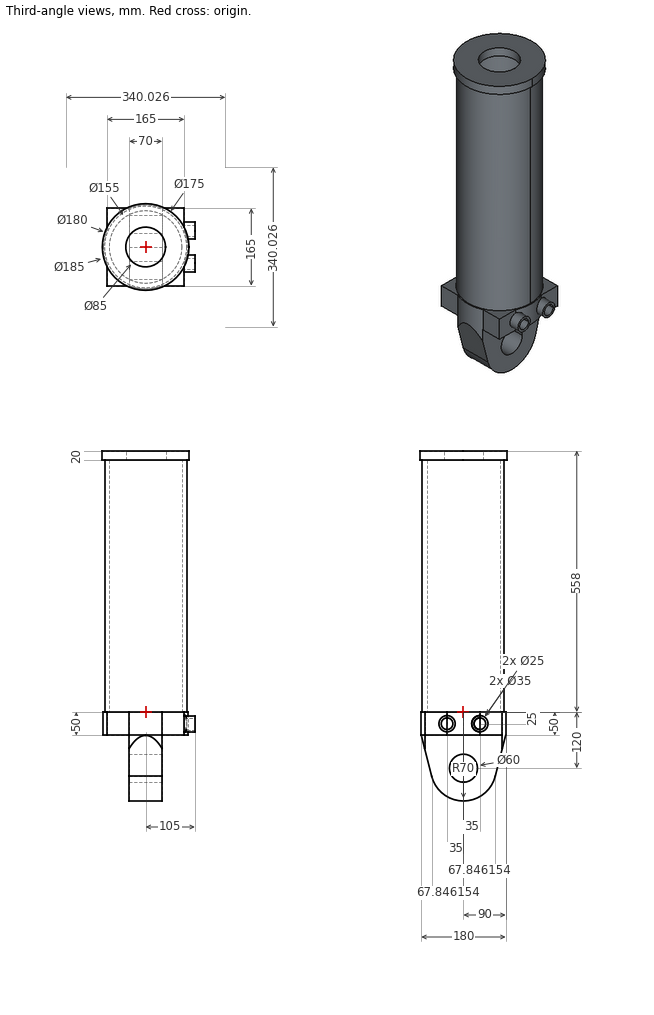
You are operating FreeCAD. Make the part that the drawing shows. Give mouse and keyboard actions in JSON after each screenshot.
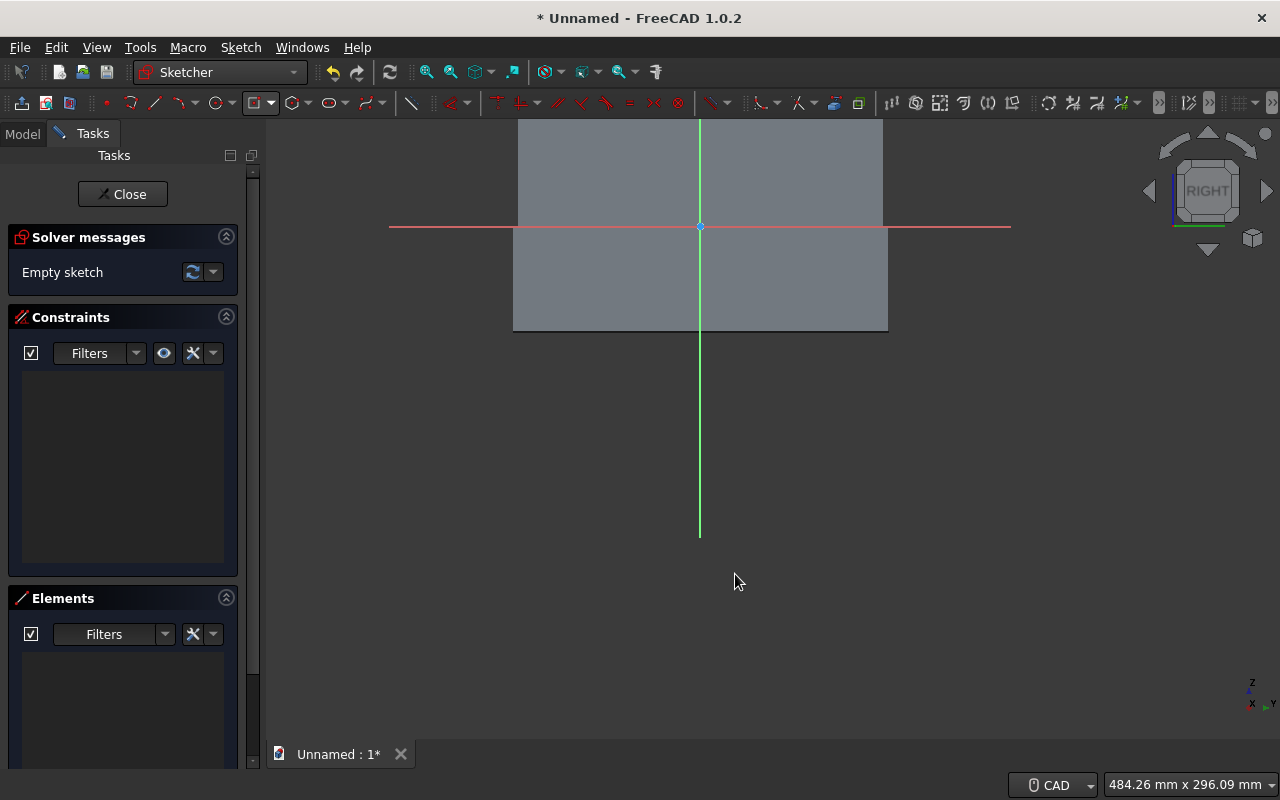
{"action": "left_click", "coordinate": [132, 104]}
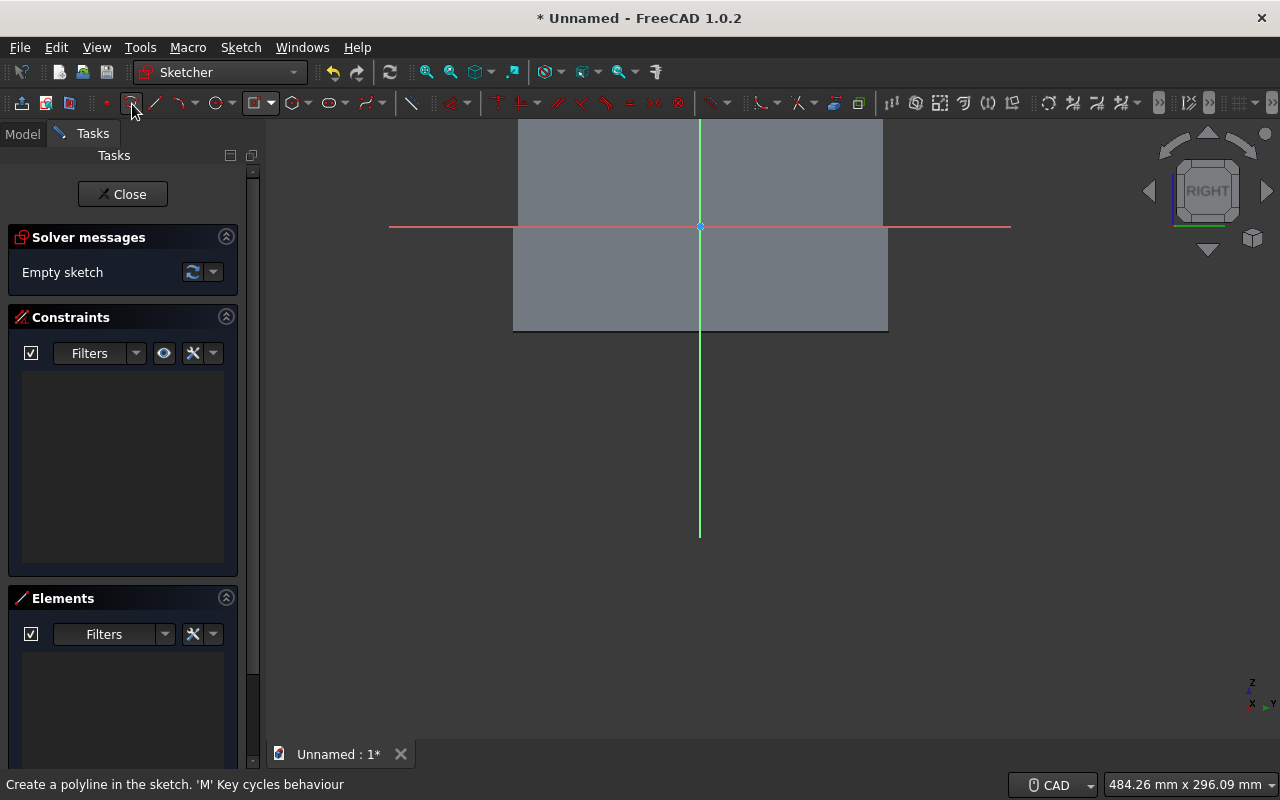
{"action": "left_click", "coordinate": [842, 514]}
{"action": "left_click", "coordinate": [889, 332]}
{"action": "left_click", "coordinate": [512, 332]}
{"action": "left_click", "coordinate": [558, 514]}
{"action": "right_click", "coordinate": [558, 514]}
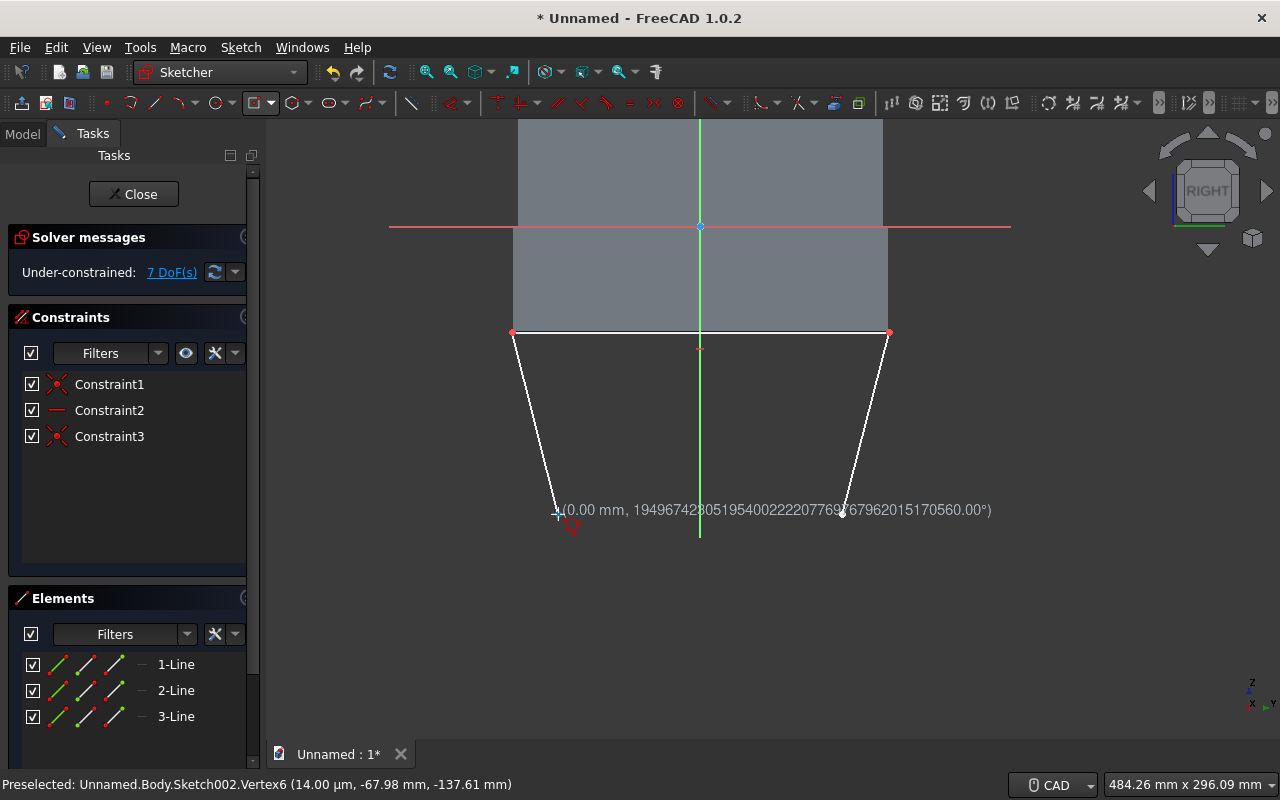
{"action": "left_click", "coordinate": [180, 104]}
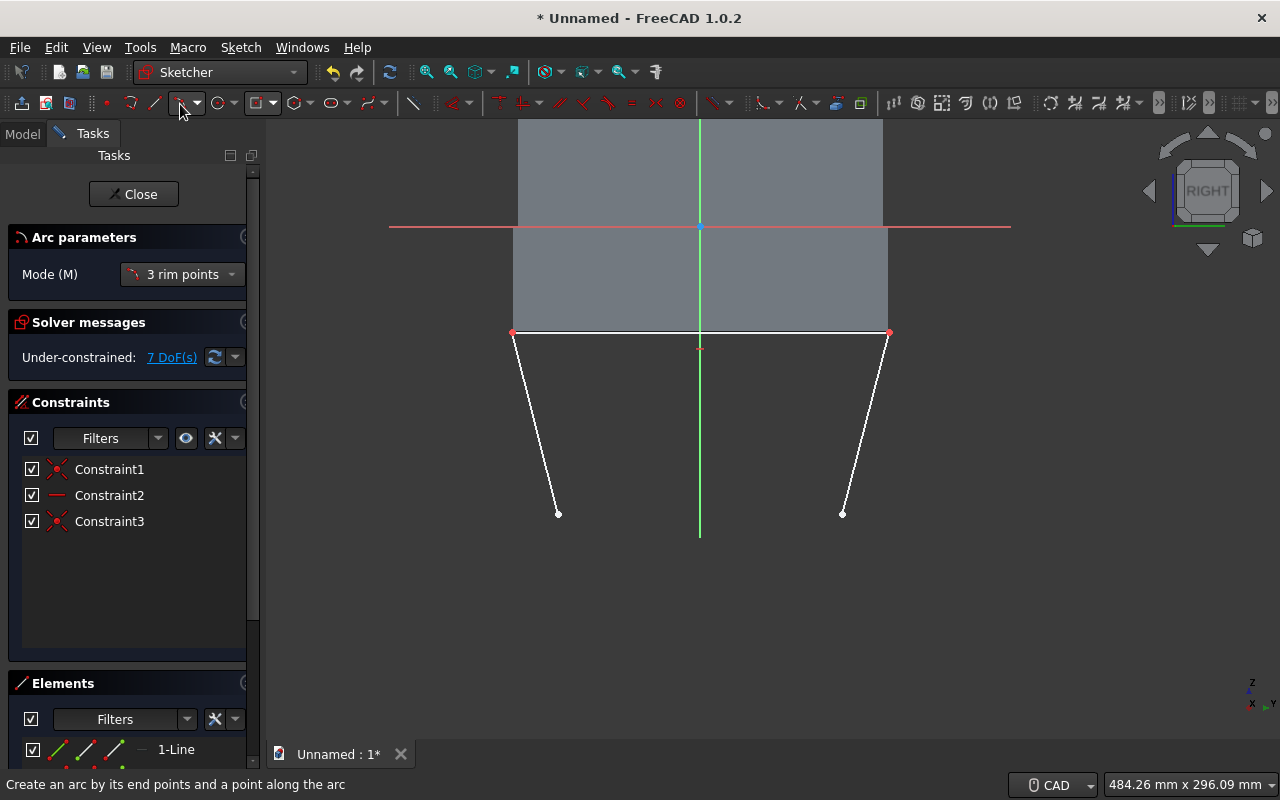
{"action": "left_click", "coordinate": [558, 515]}
{"action": "left_click", "coordinate": [842, 515]}
{"action": "left_click", "coordinate": [662, 620]}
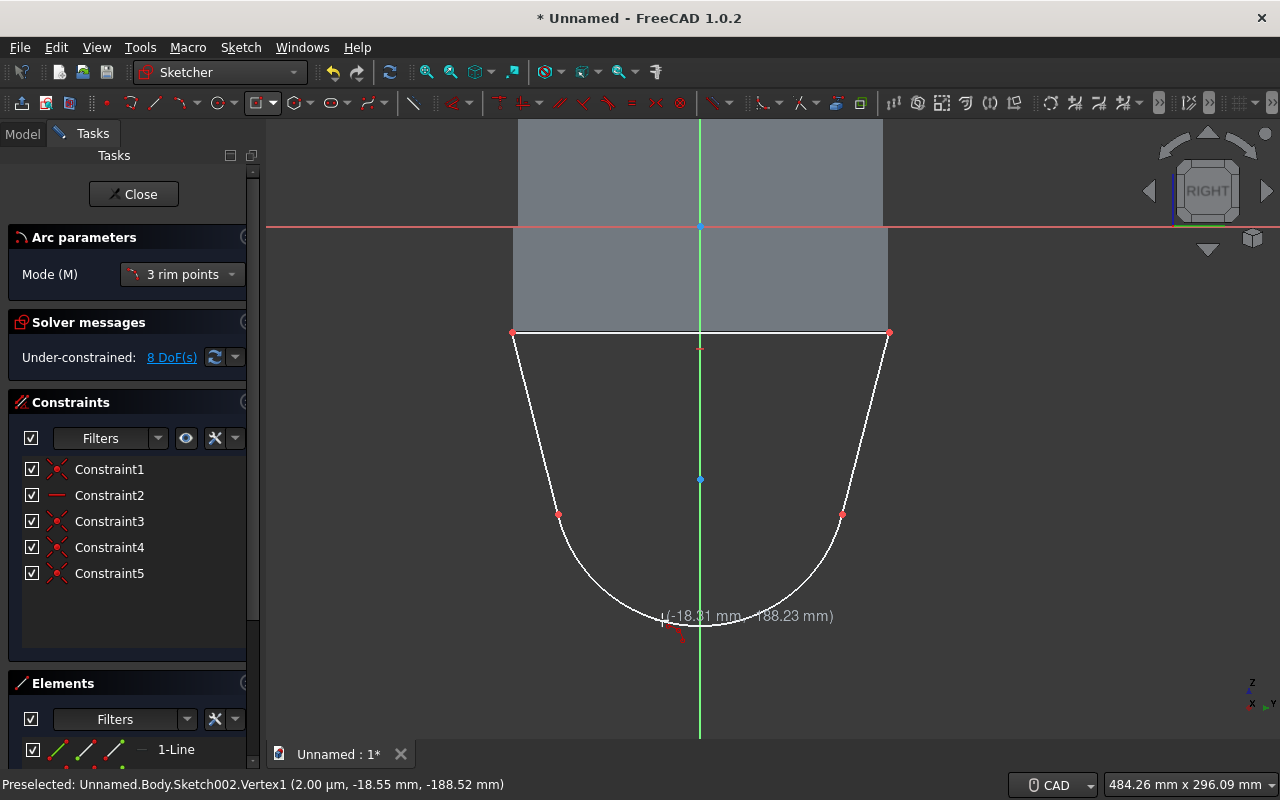
{"action": "key", "text": "g c"}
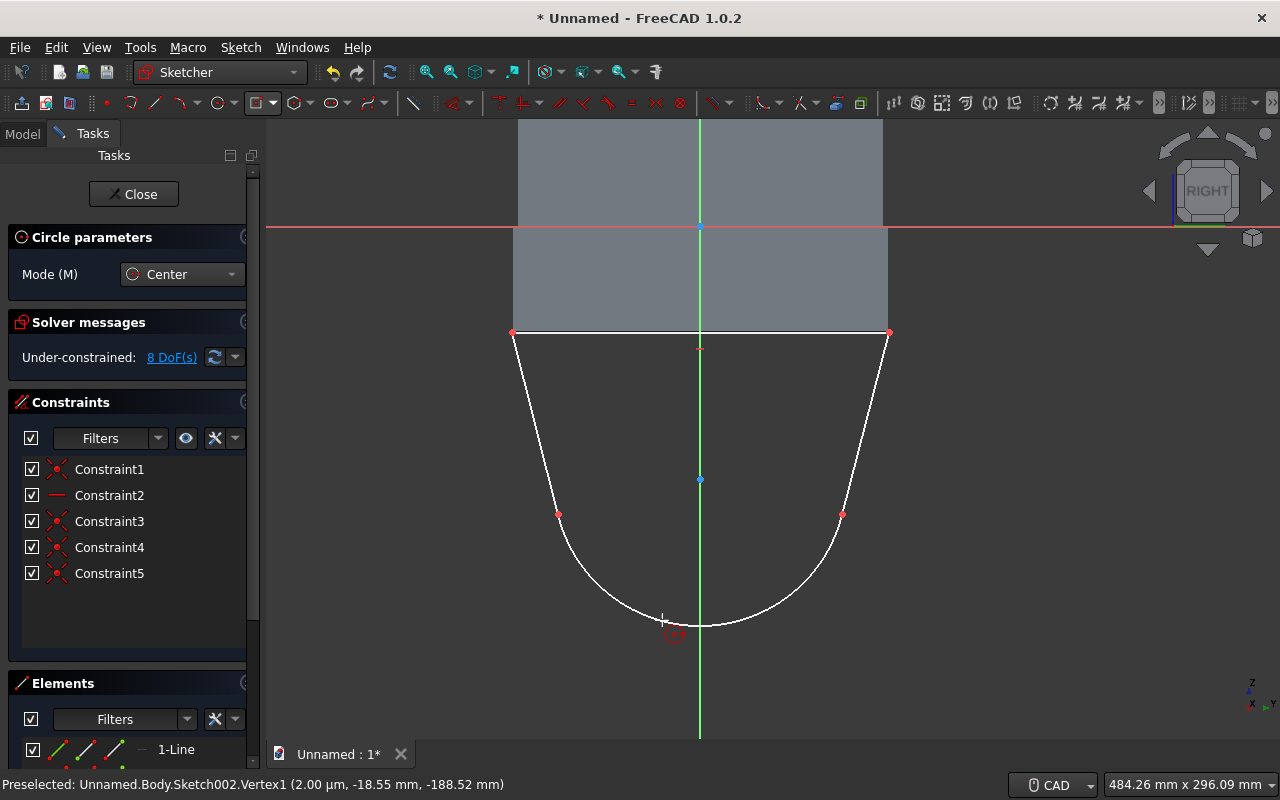
{"action": "left_click", "coordinate": [700, 478]}
{"action": "left_click", "coordinate": [745, 434]}
{"action": "key", "text": "Escape"}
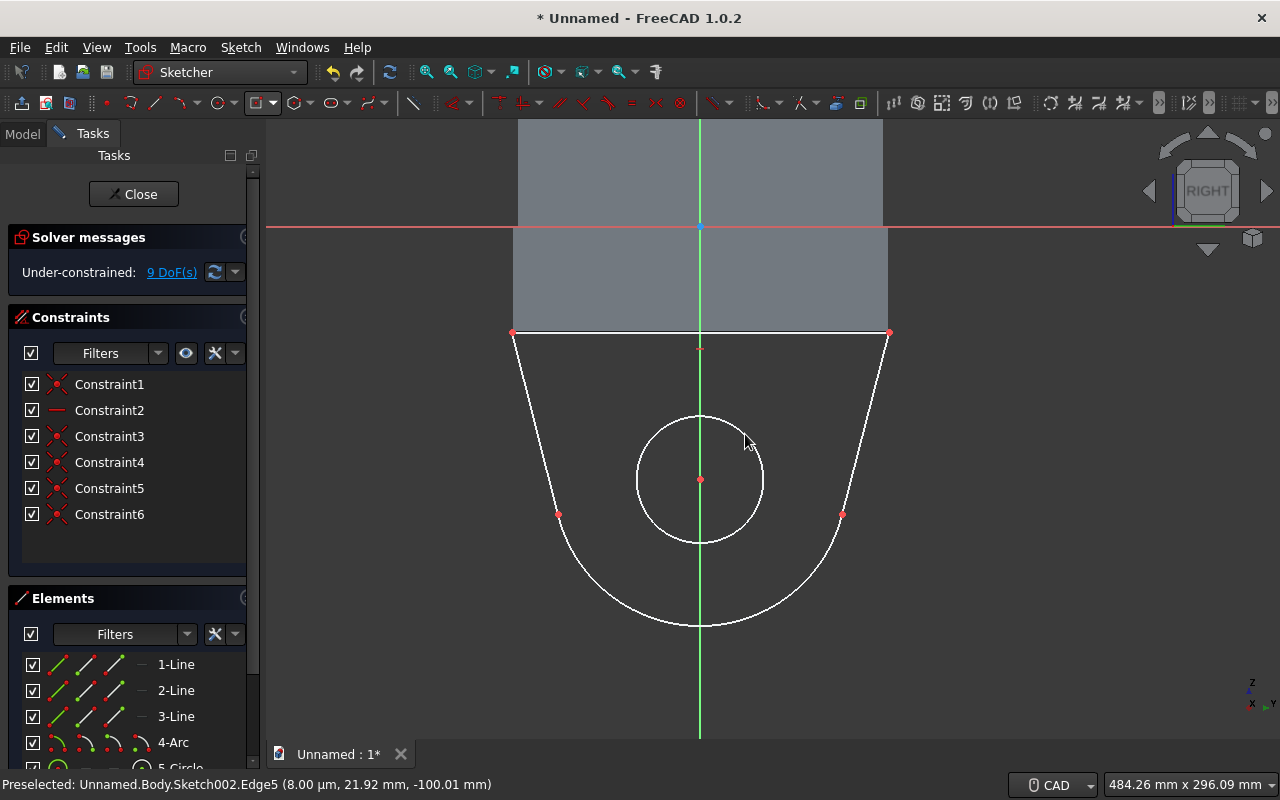
{"action": "left_click", "coordinate": [700, 480]}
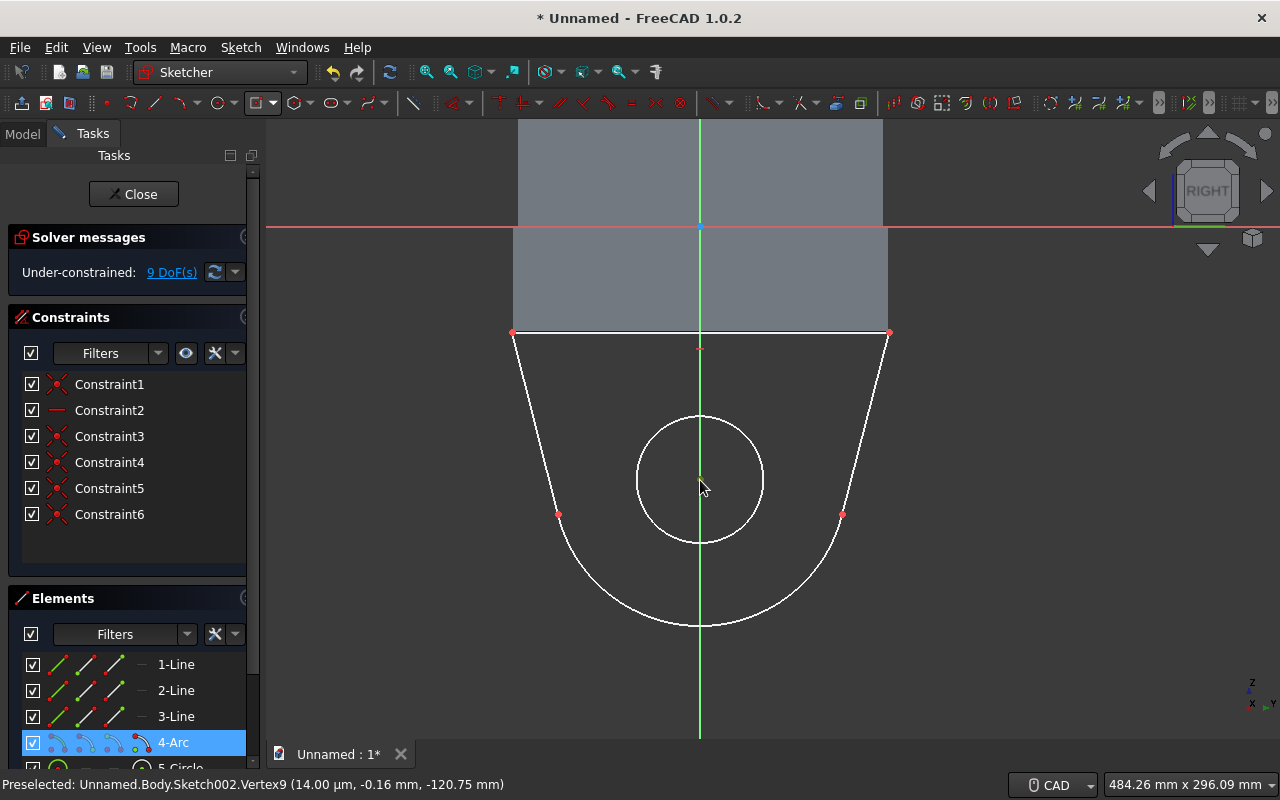
{"action": "left_click", "coordinate": [700, 671]}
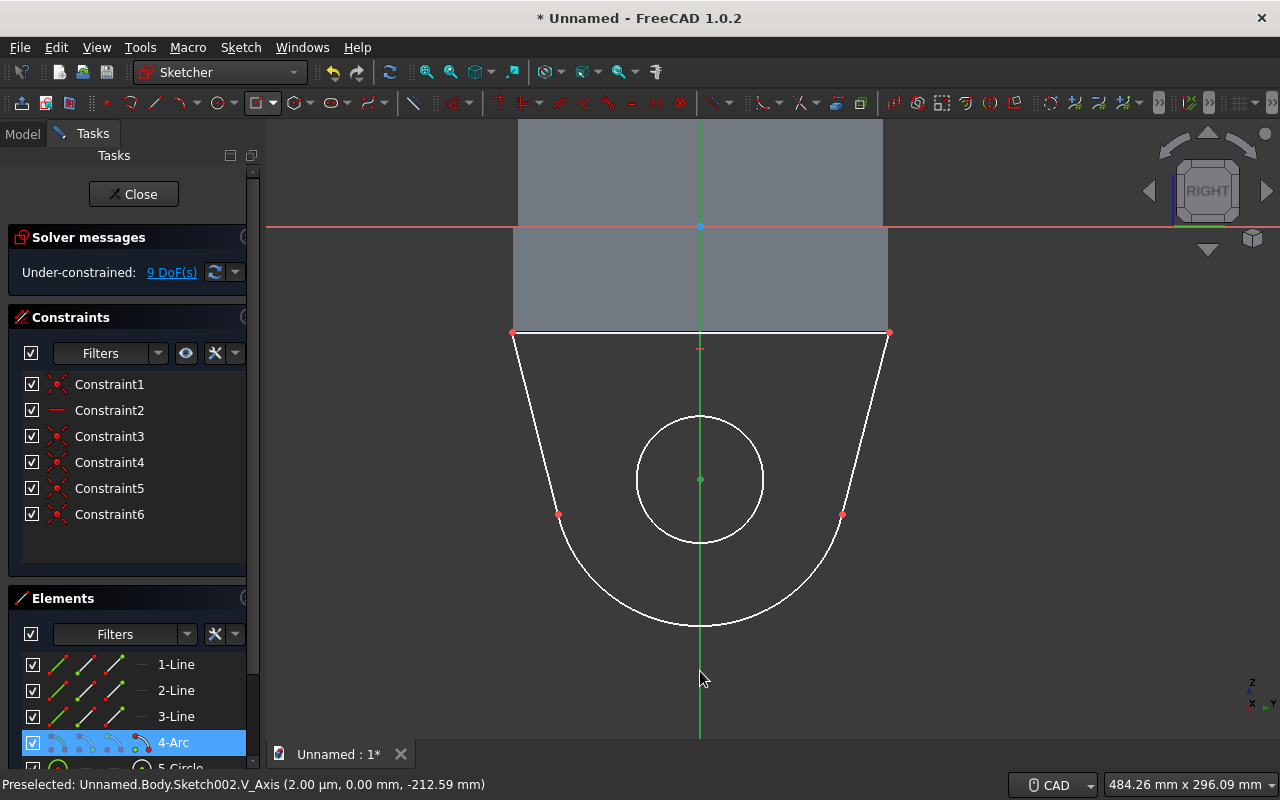
{"action": "left_click", "coordinate": [500, 104]}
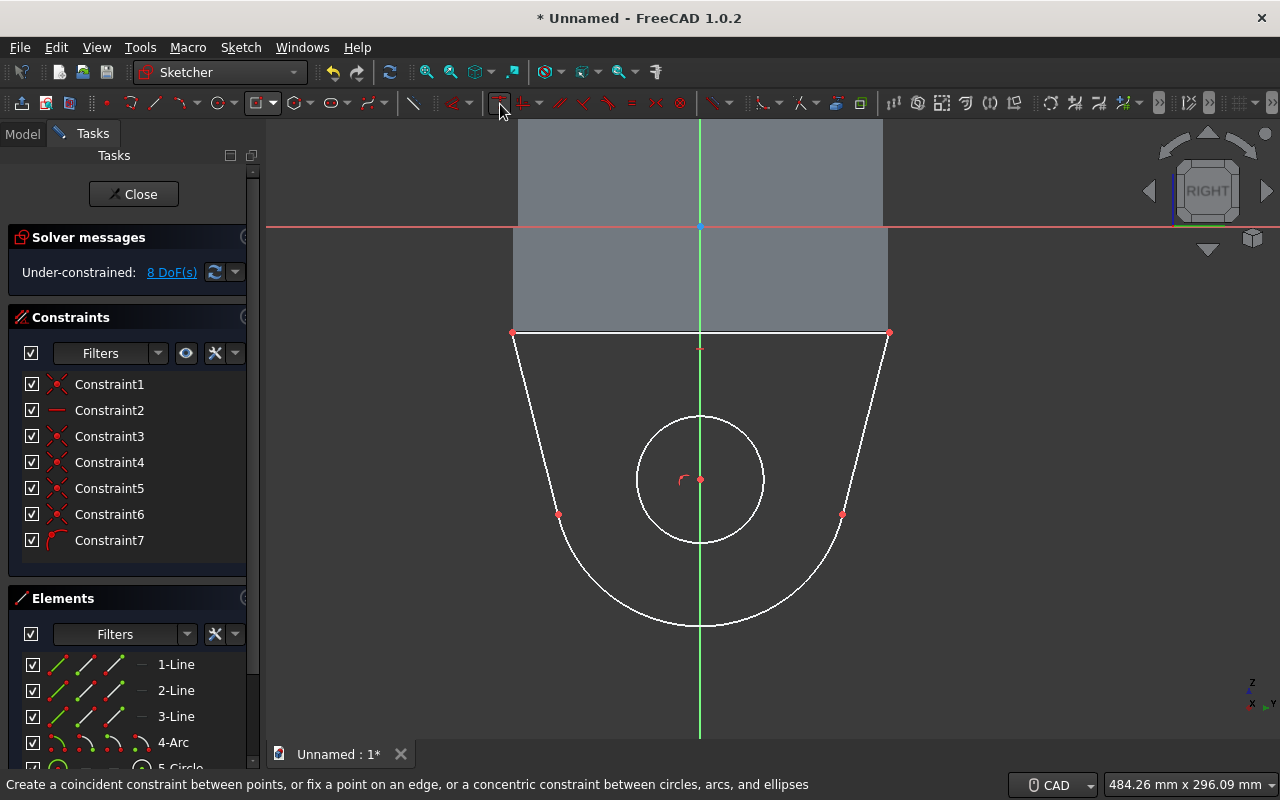
{"action": "left_click", "coordinate": [452, 104]}